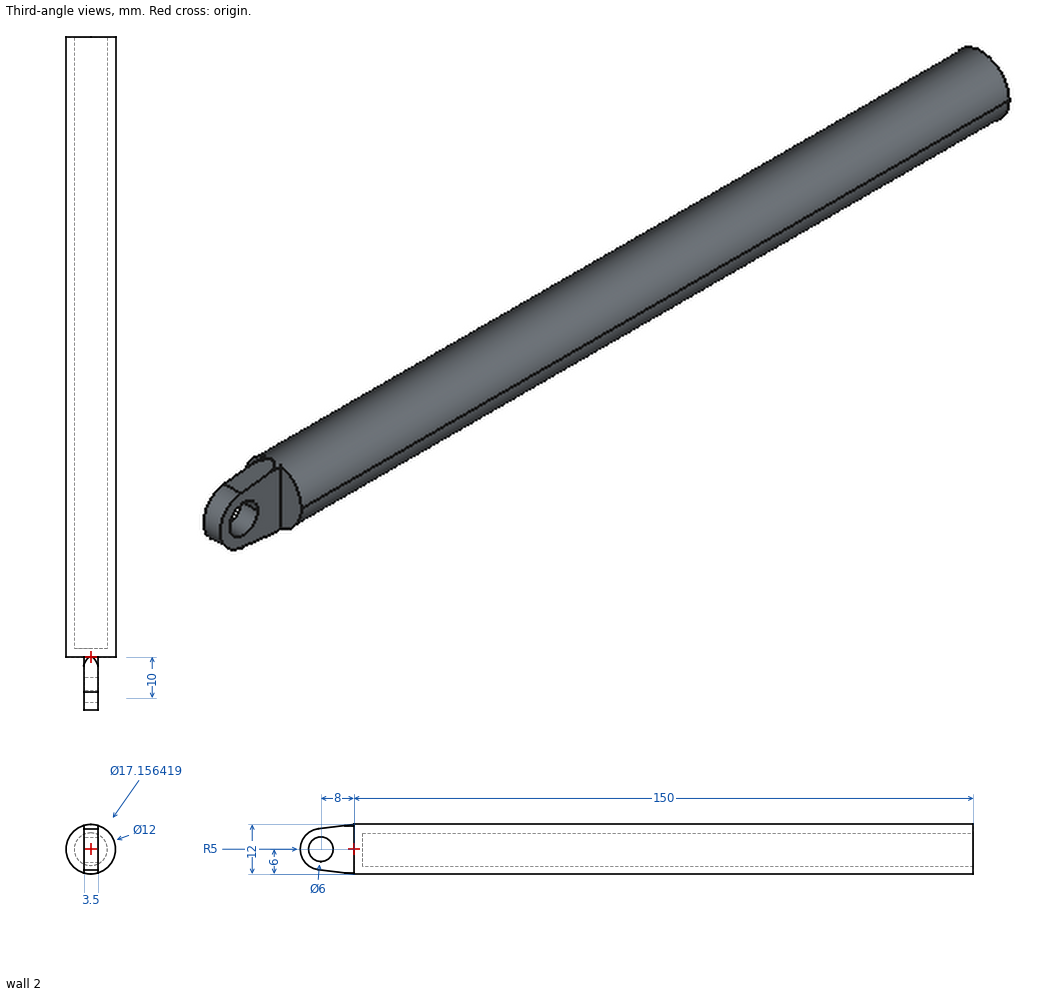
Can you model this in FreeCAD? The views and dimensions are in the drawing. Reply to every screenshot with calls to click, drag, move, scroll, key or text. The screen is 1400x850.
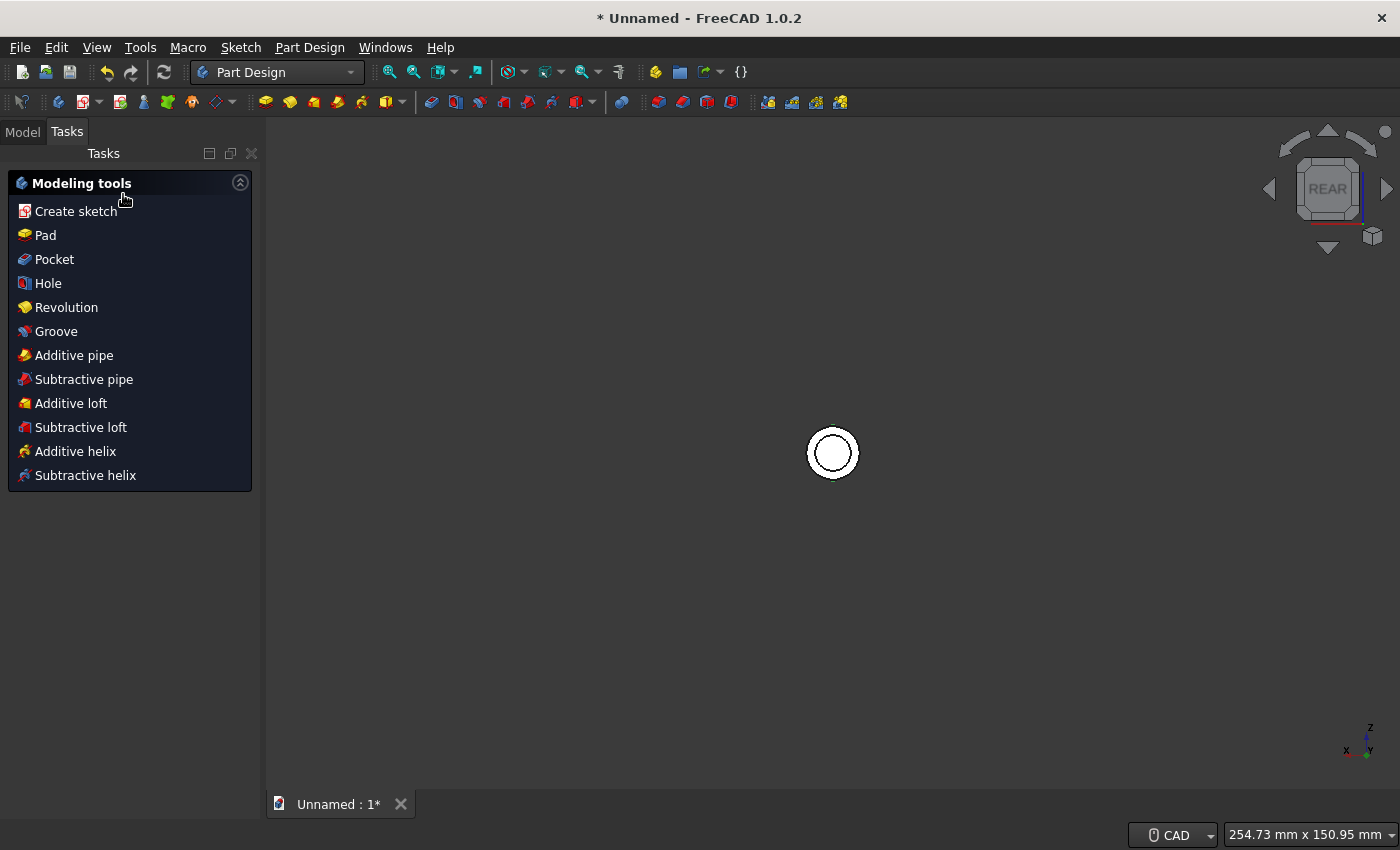
click(266, 102)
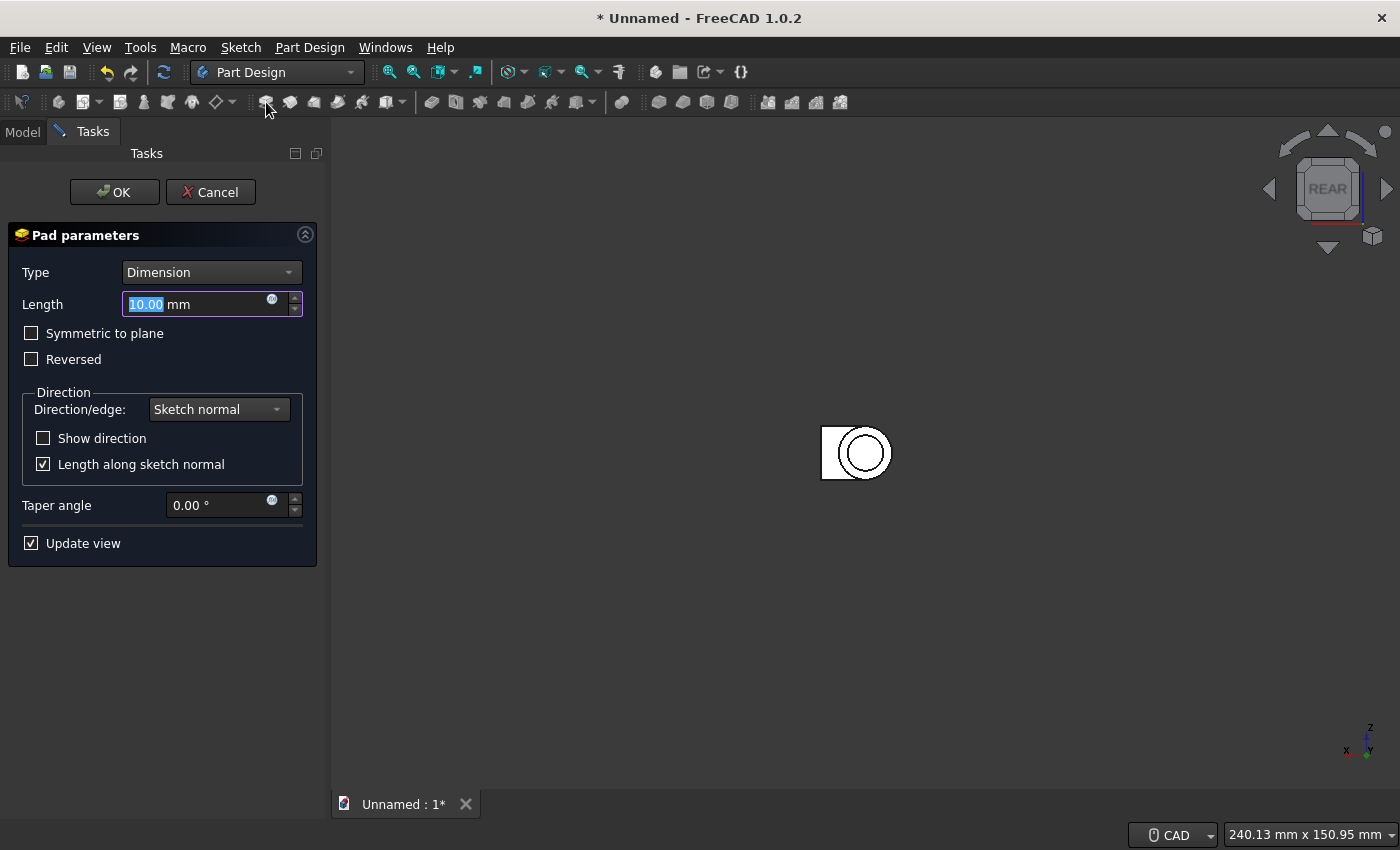
text(3.5)
key(Tab)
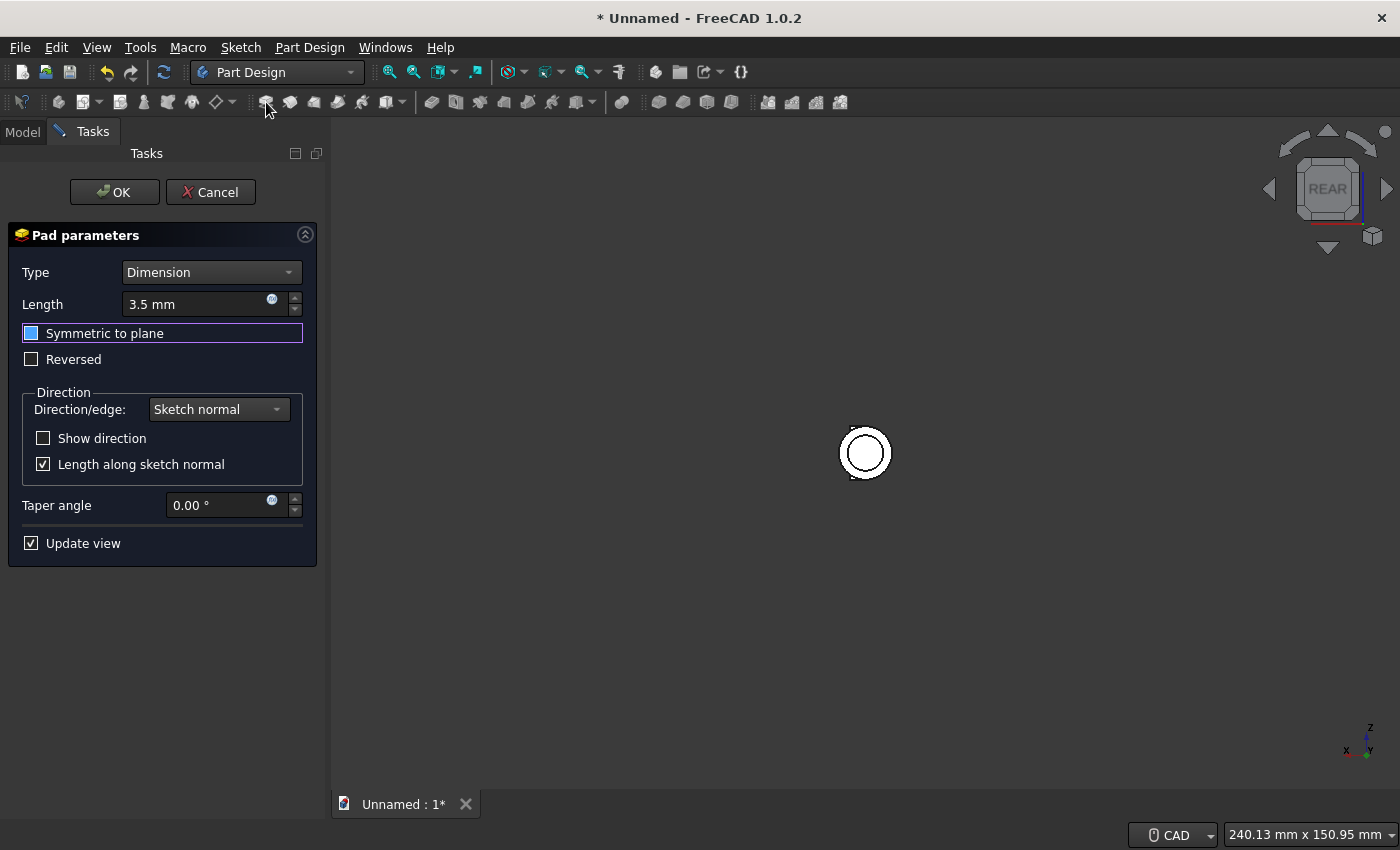
click(30, 333)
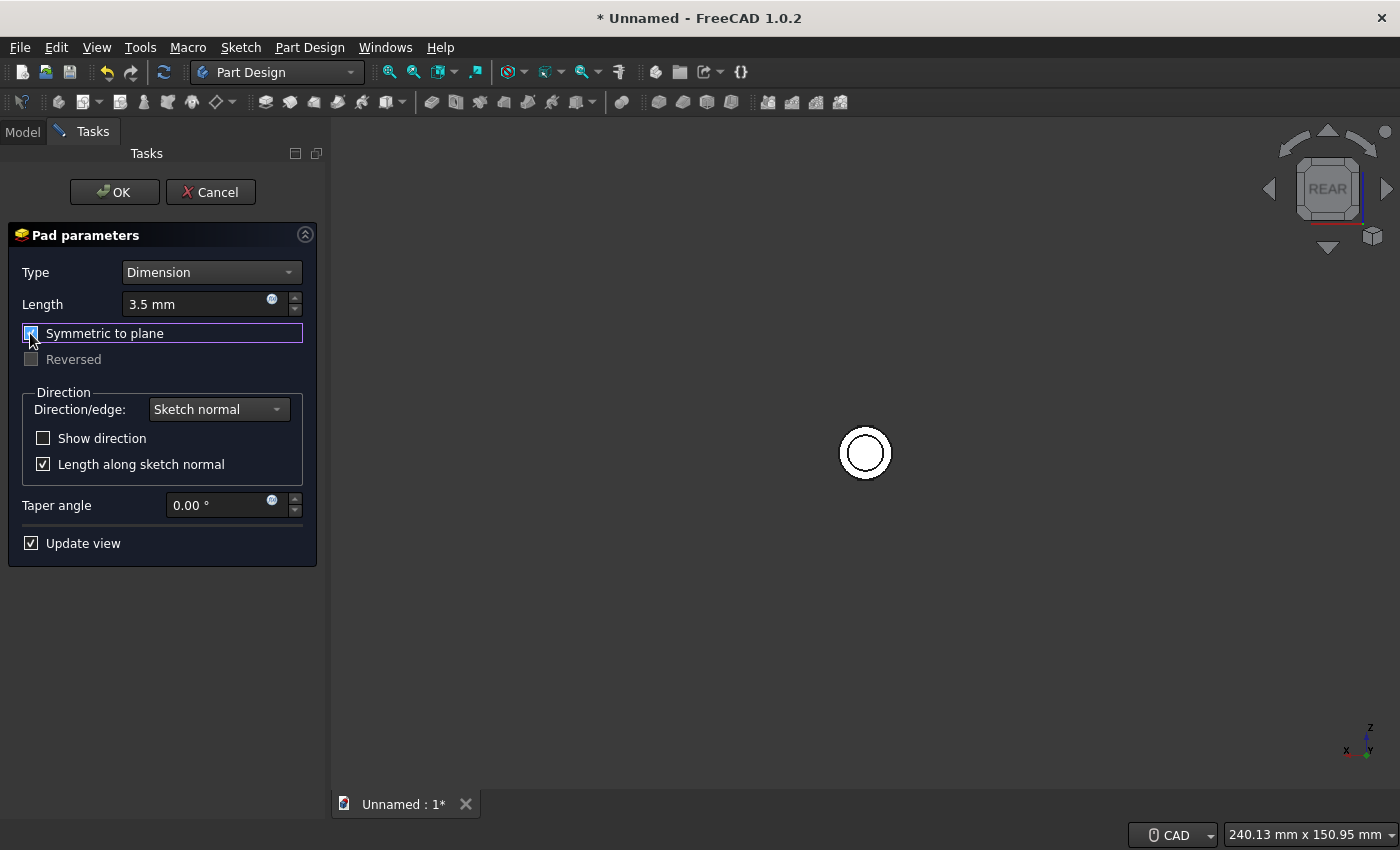
click(115, 192)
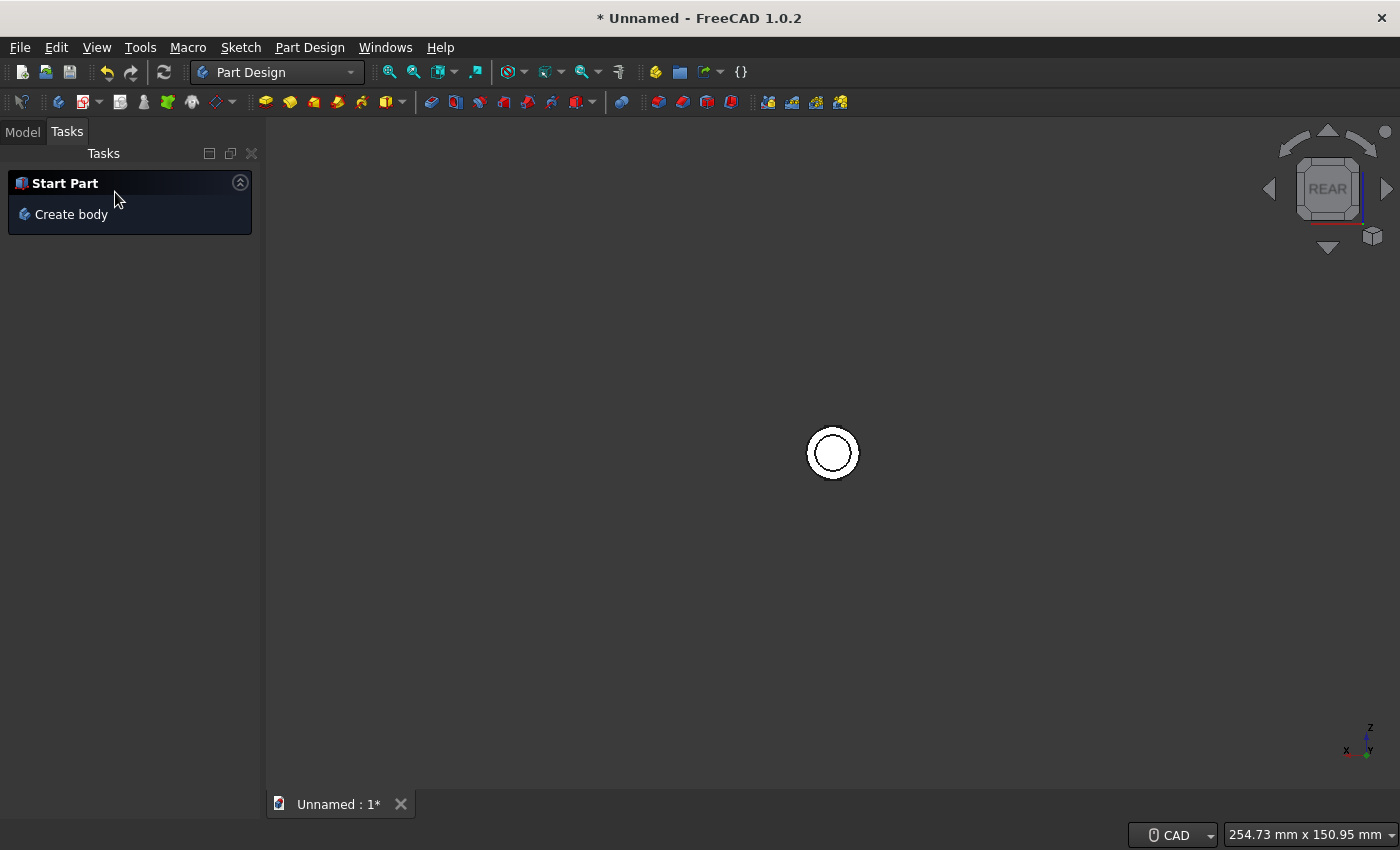
click(390, 72)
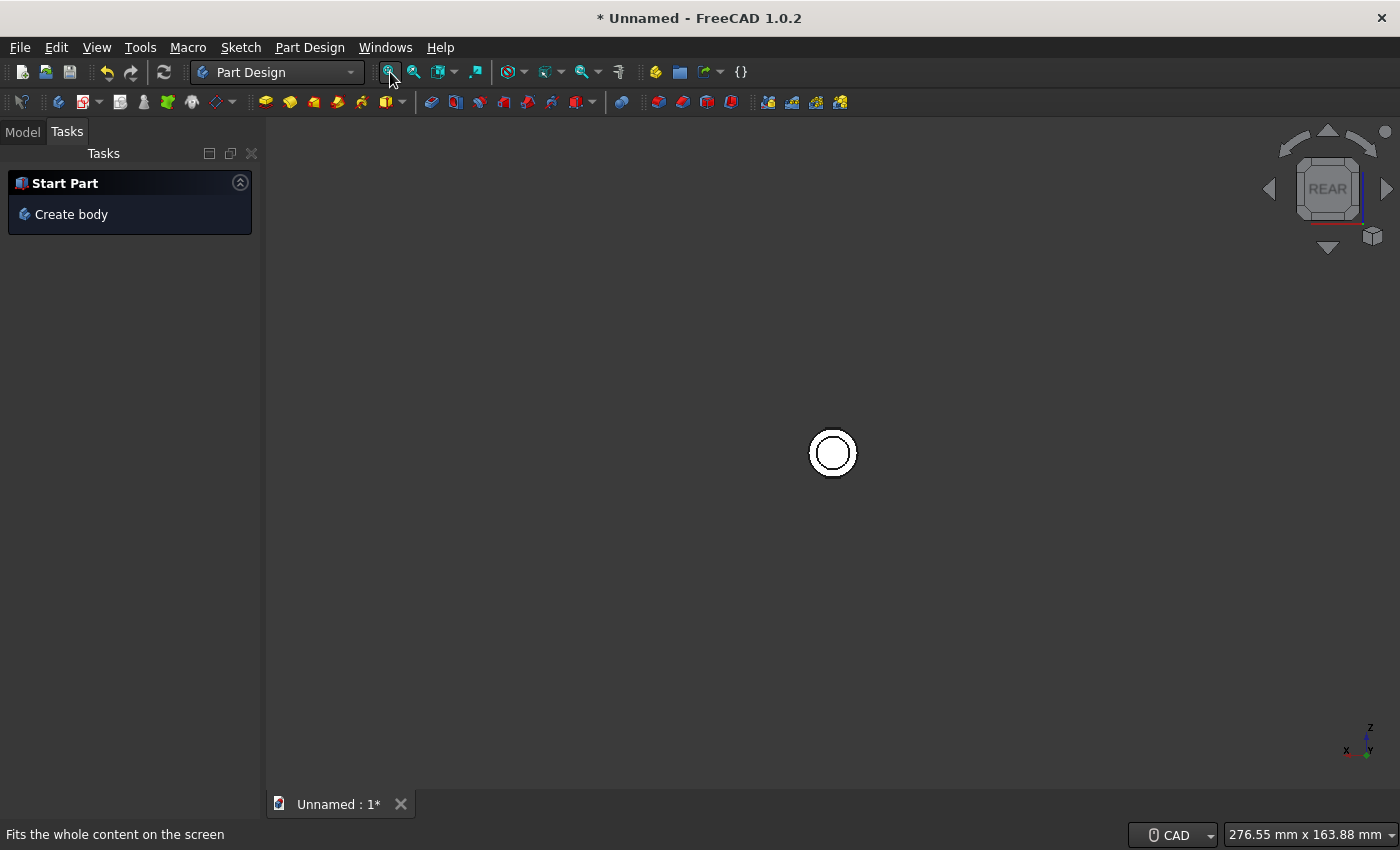
click(23, 131)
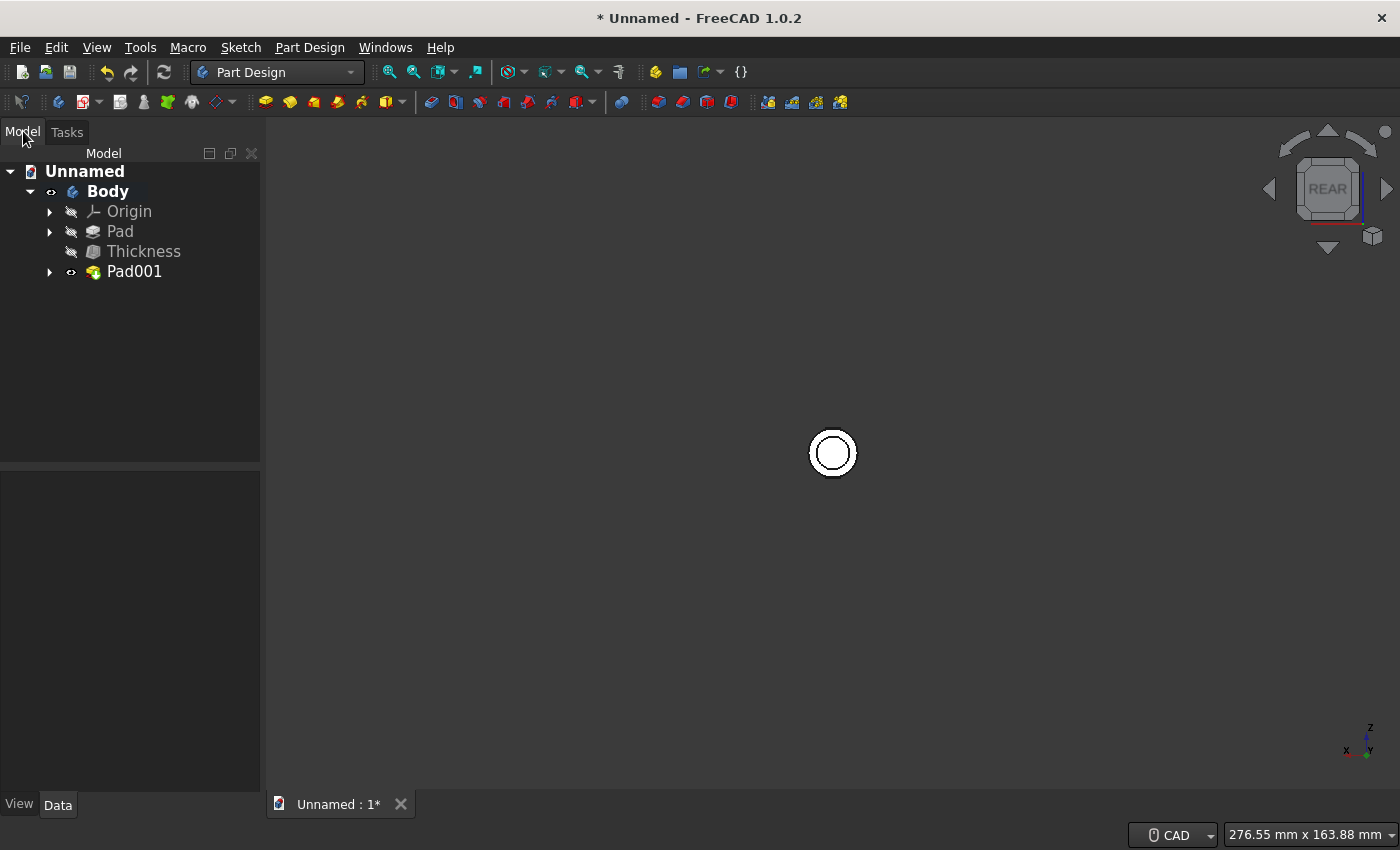
click(50, 212)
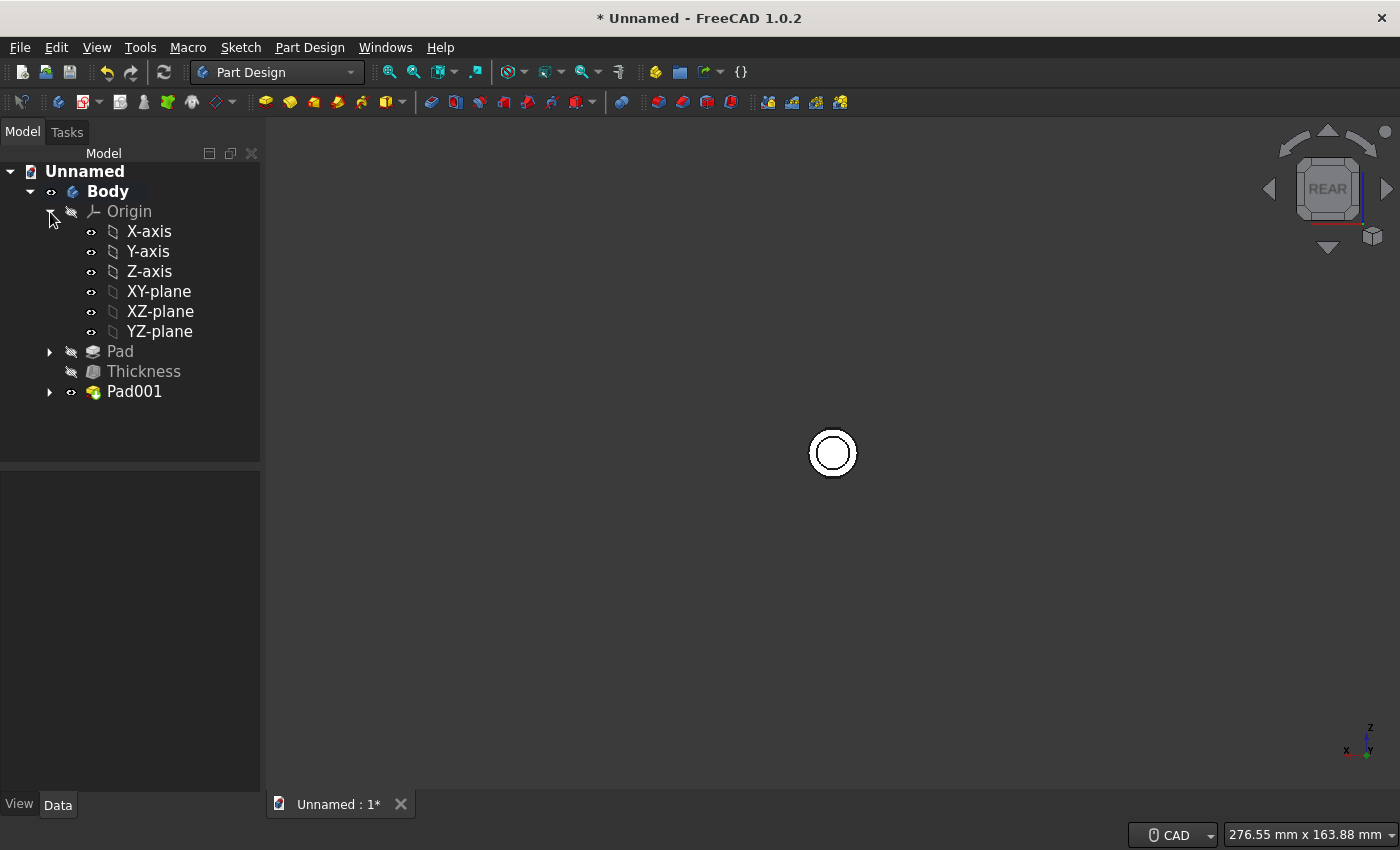
click(136, 312)